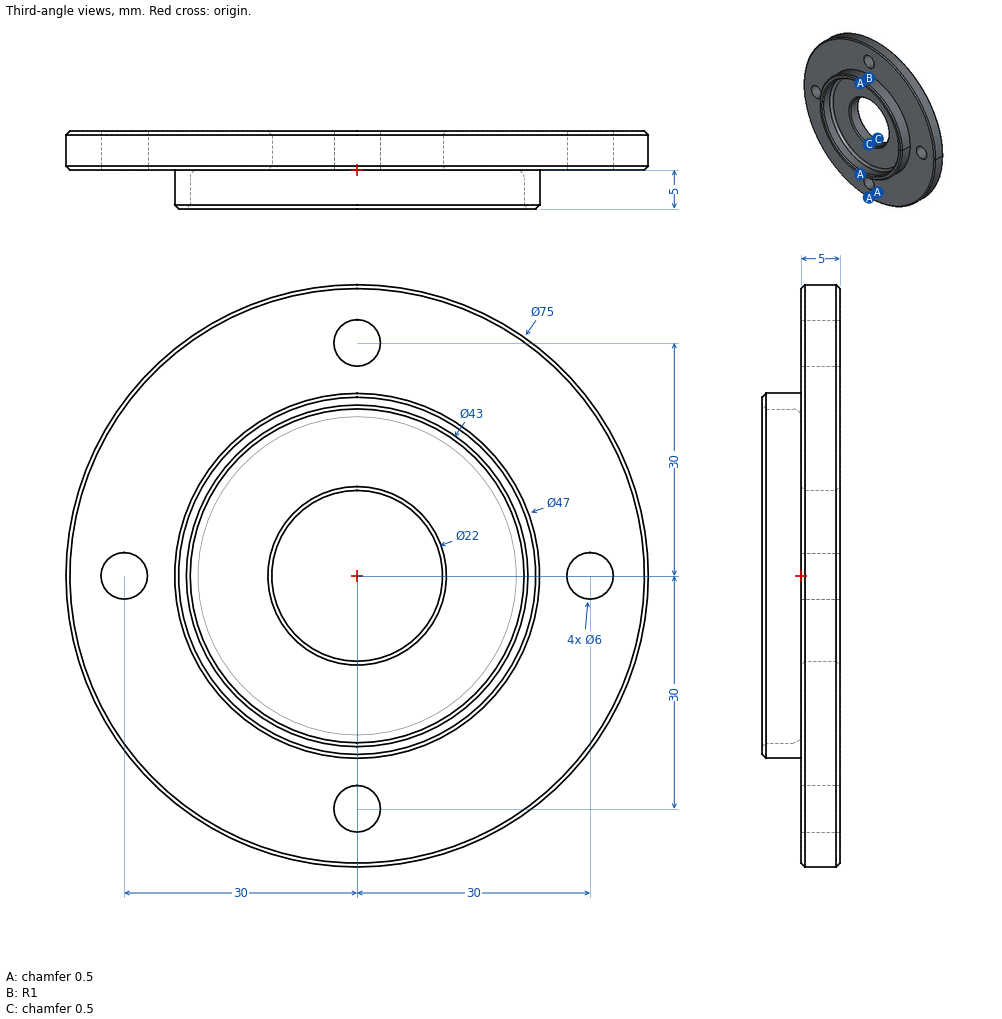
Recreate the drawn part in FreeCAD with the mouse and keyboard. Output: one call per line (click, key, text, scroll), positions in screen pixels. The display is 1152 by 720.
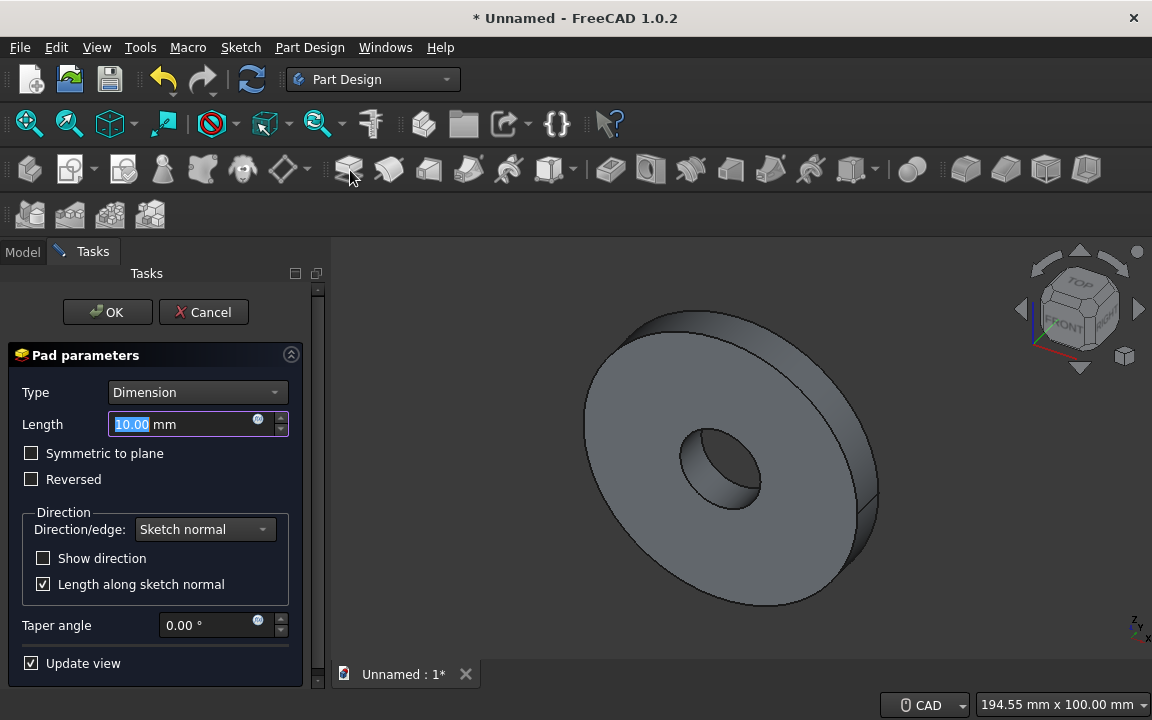
text(5)
key(Tab)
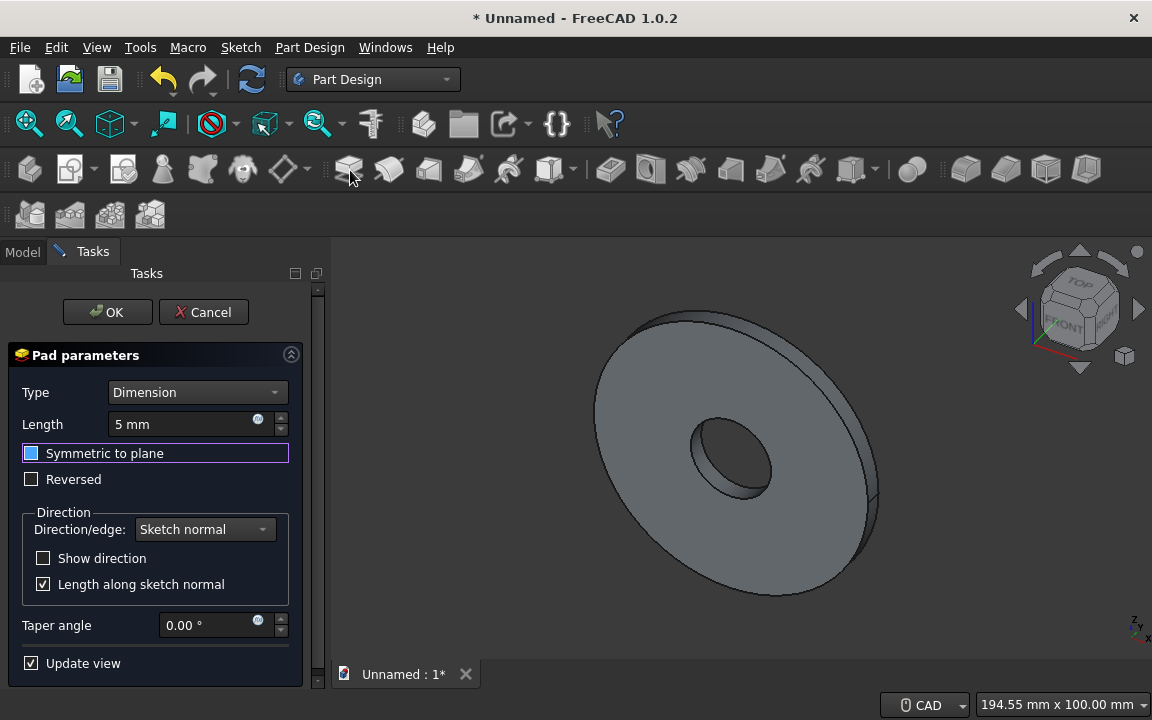
click(30, 479)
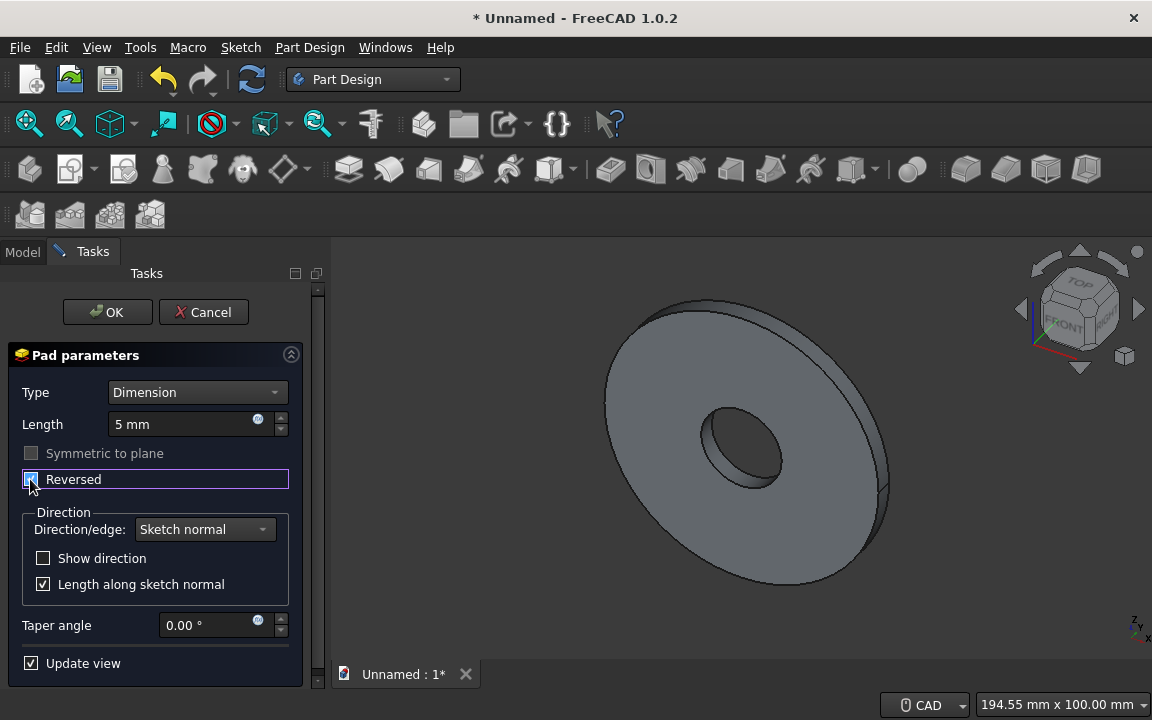
click(108, 312)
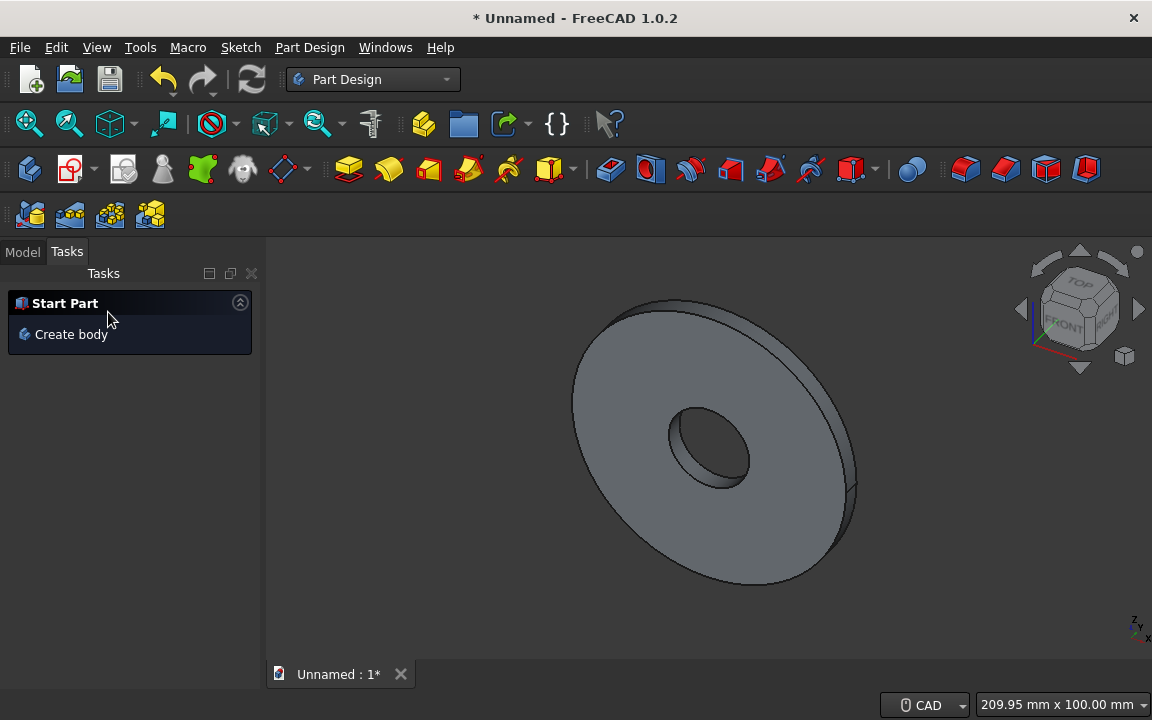
click(670, 360)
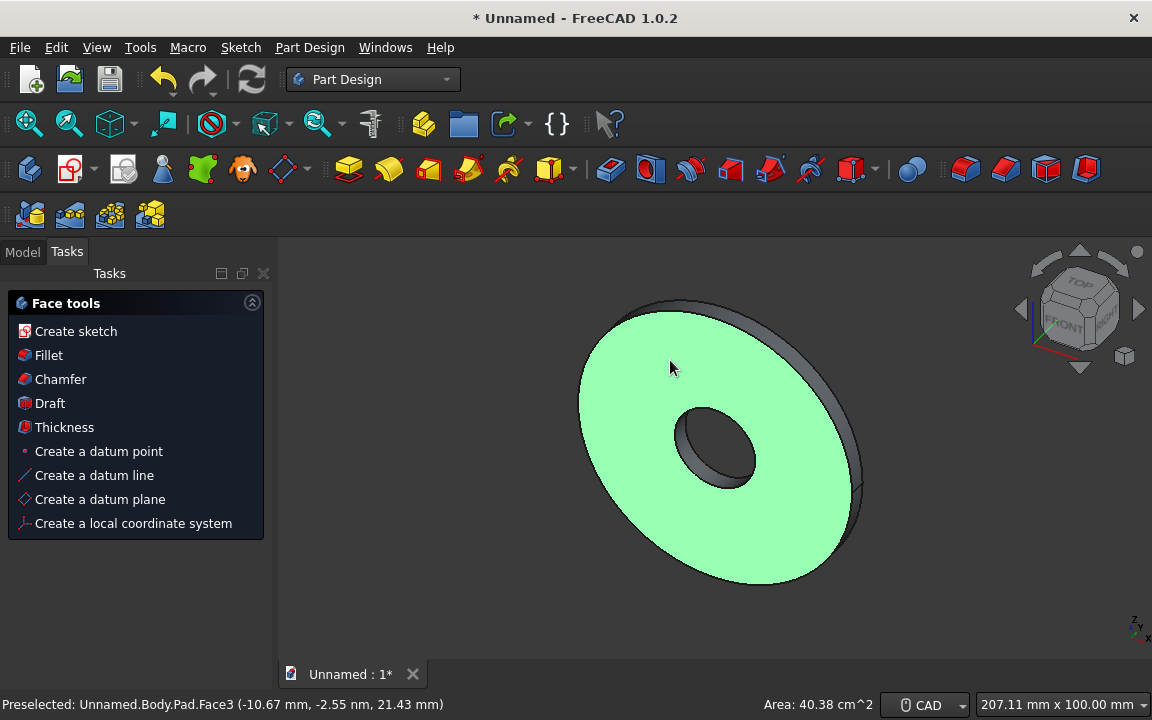
click(70, 170)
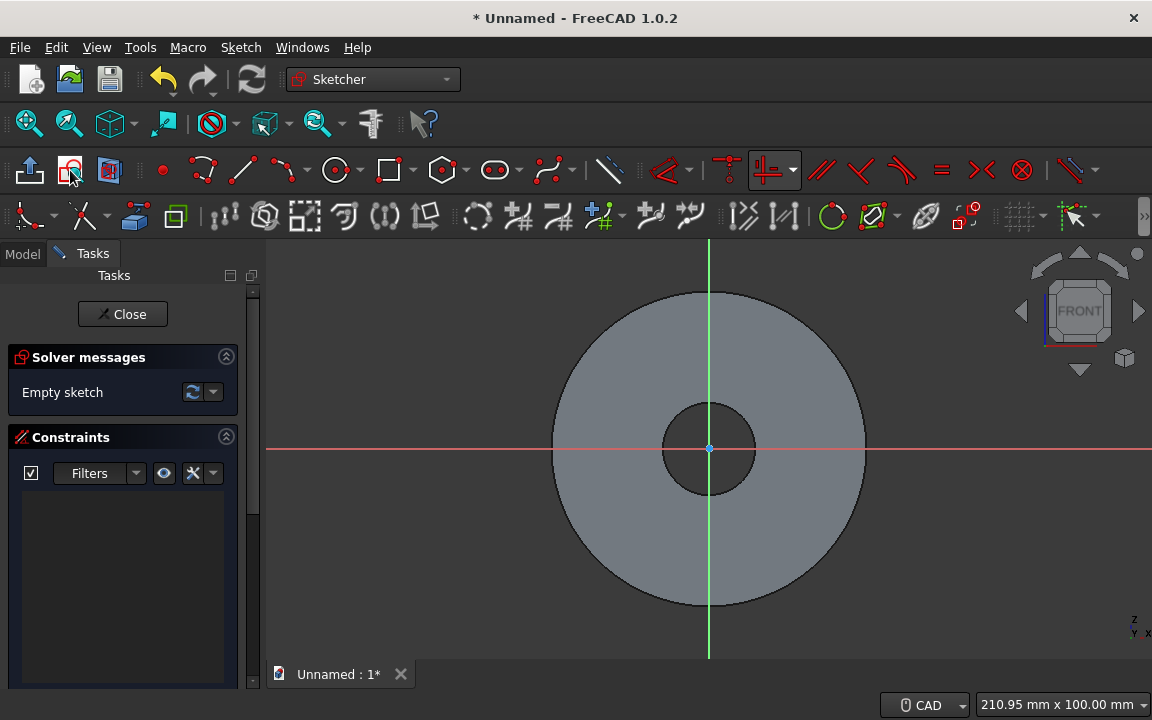
click(336, 170)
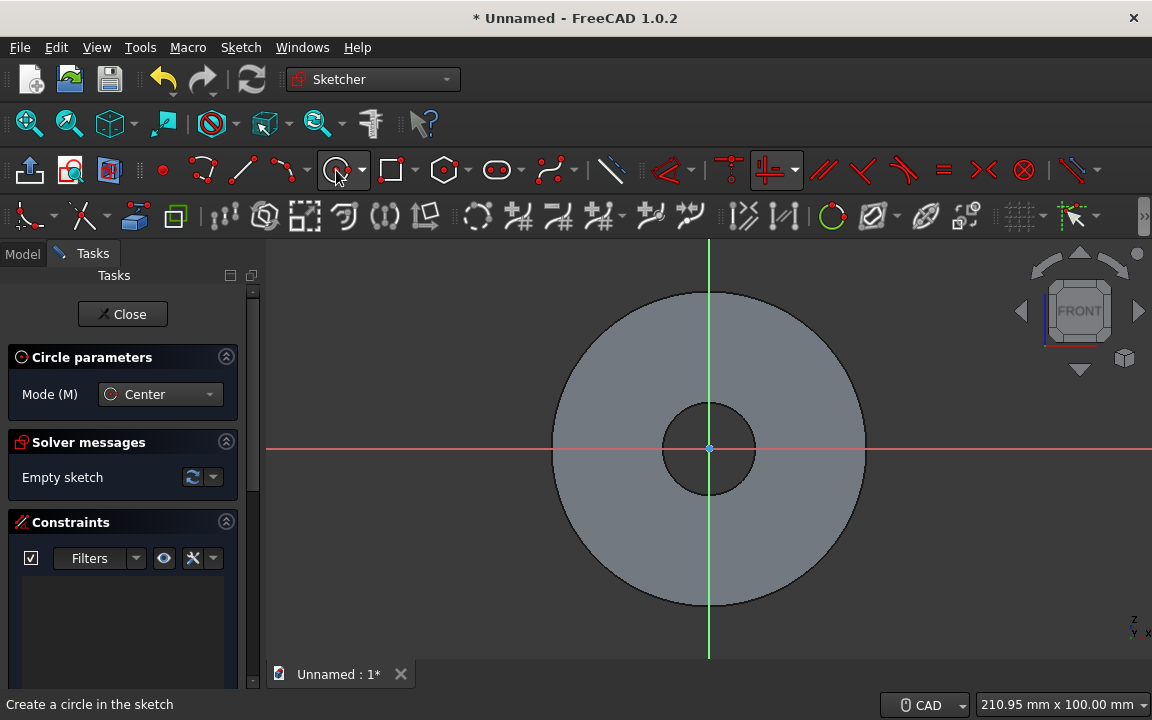
click(709, 449)
move(779, 379)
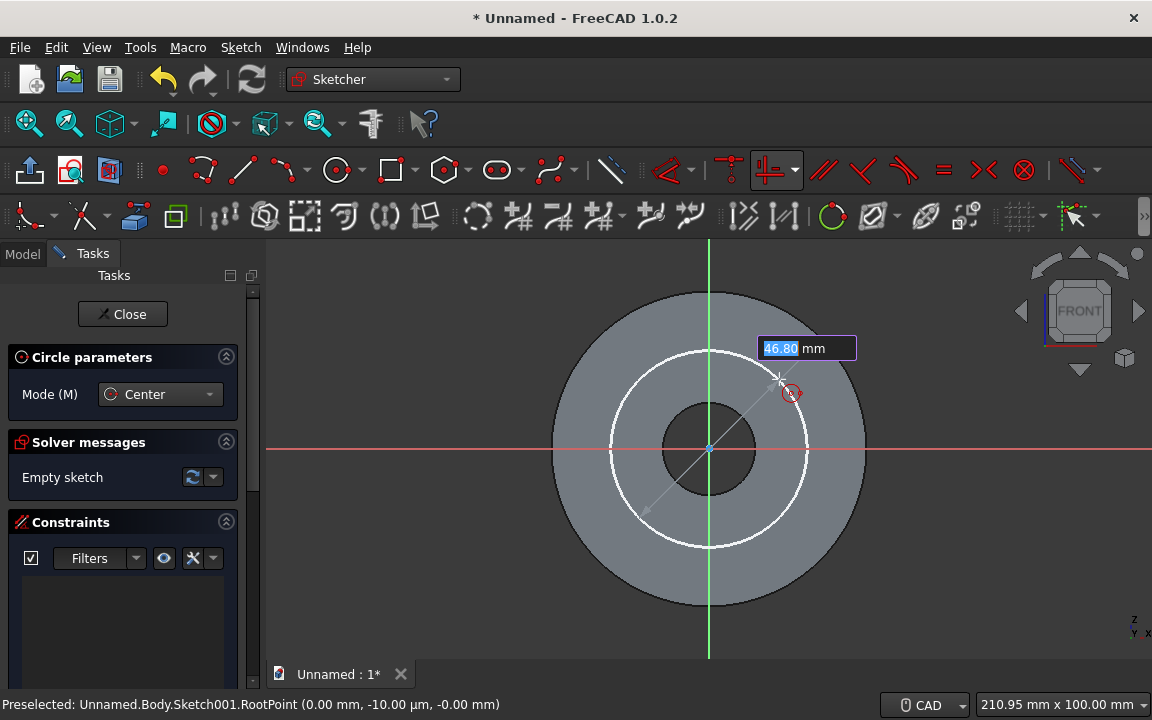
text(47)
key(Return)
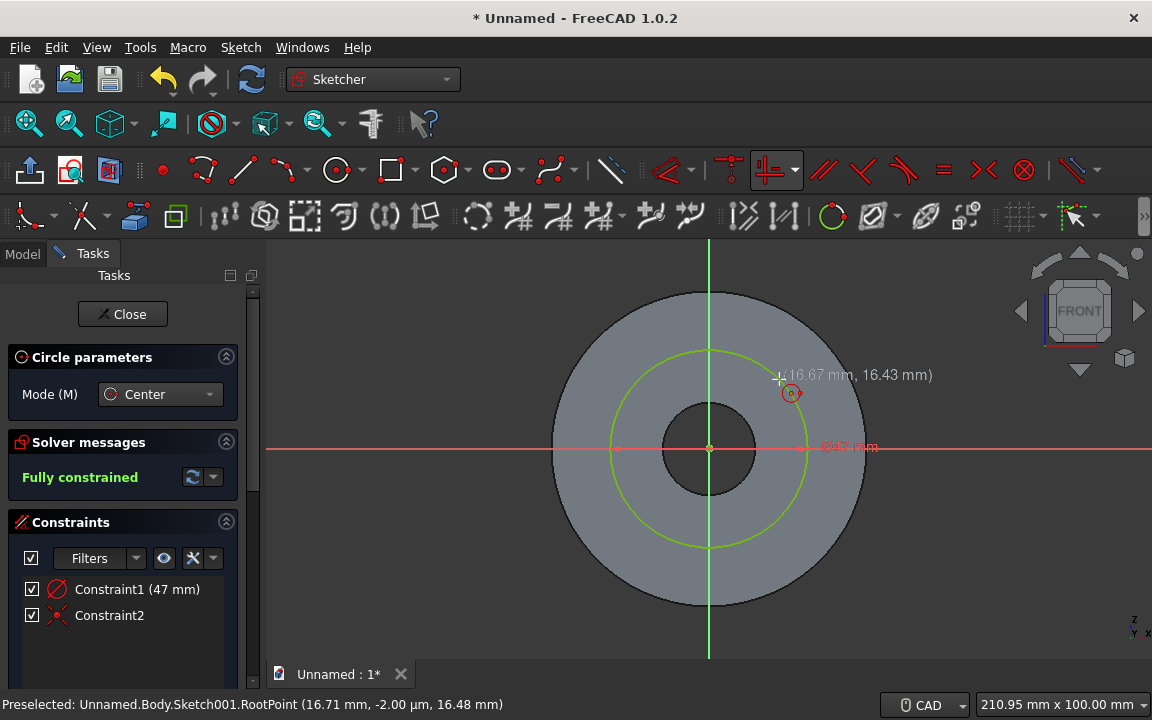
click(709, 449)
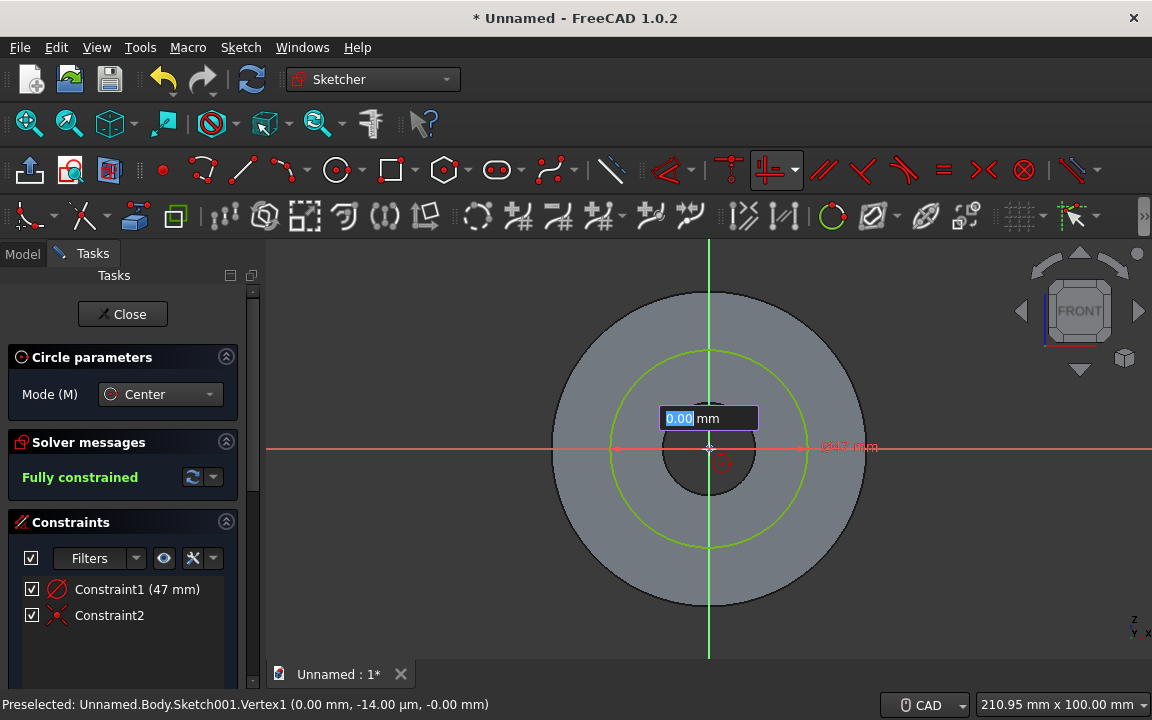
scroll(773, 385, up, 4)
move(772, 385)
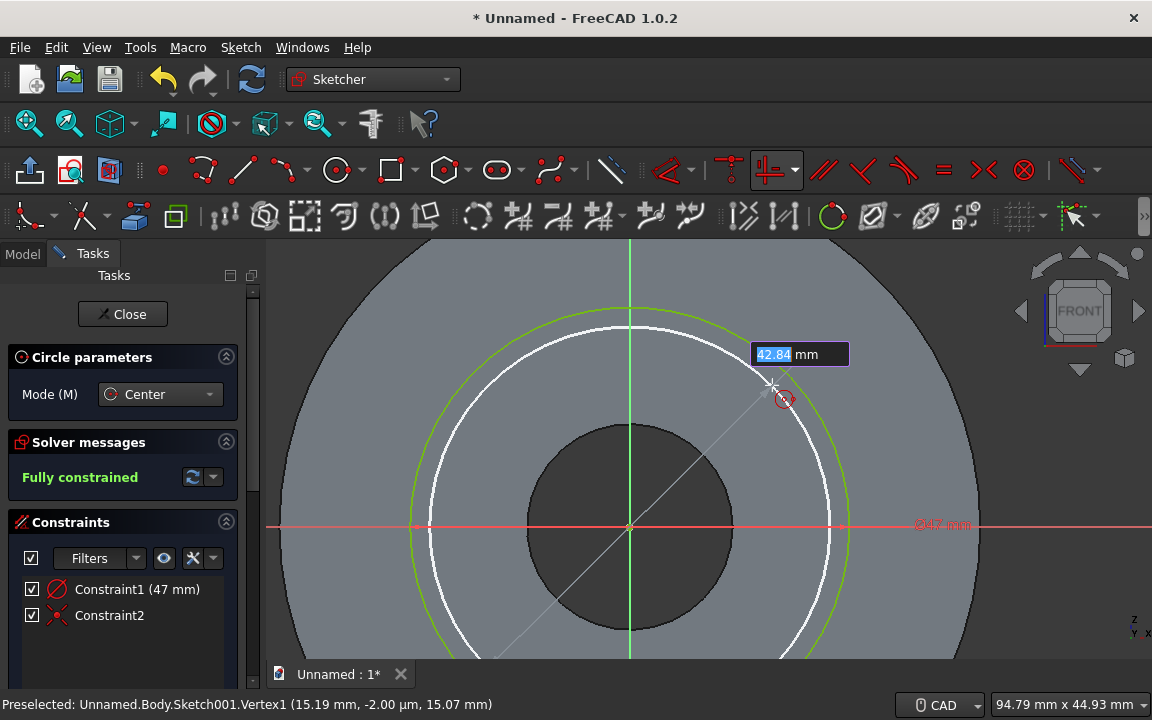
text(43)
key(Return)
key(Escape)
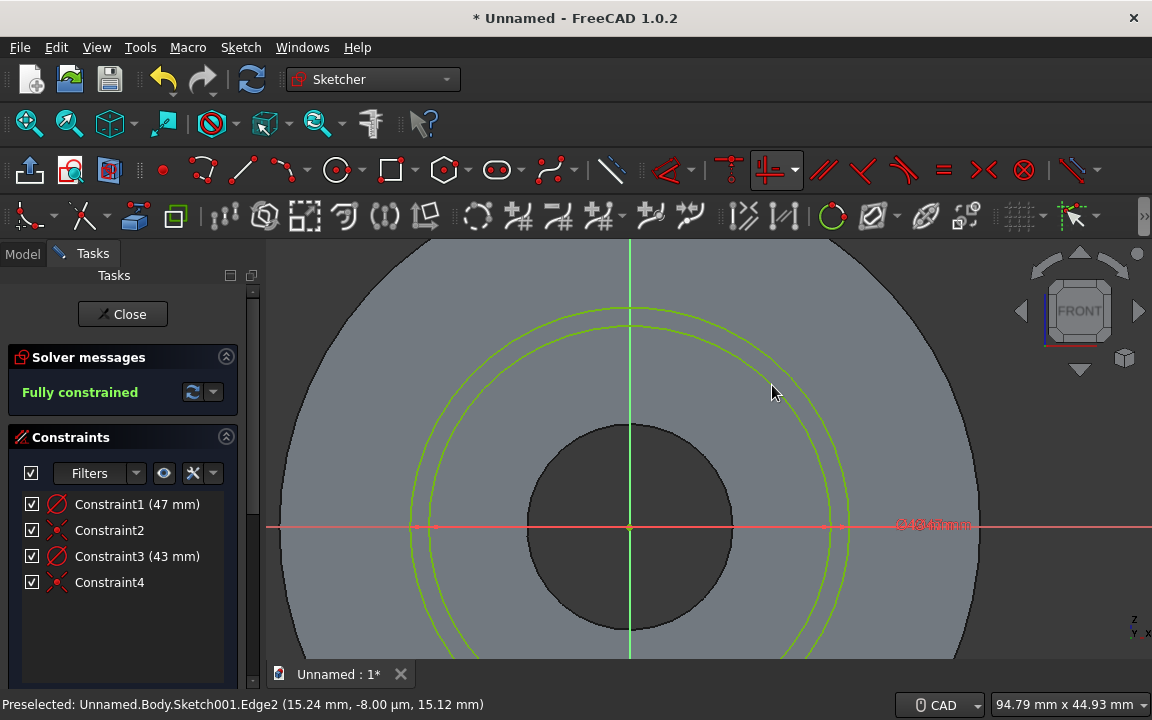
click(123, 314)